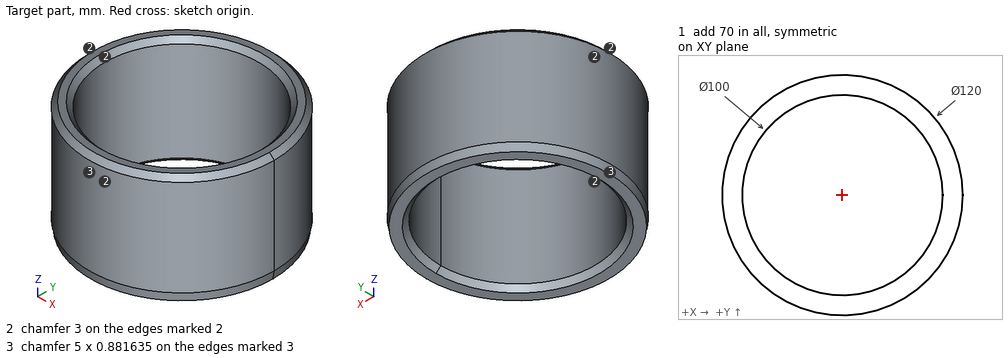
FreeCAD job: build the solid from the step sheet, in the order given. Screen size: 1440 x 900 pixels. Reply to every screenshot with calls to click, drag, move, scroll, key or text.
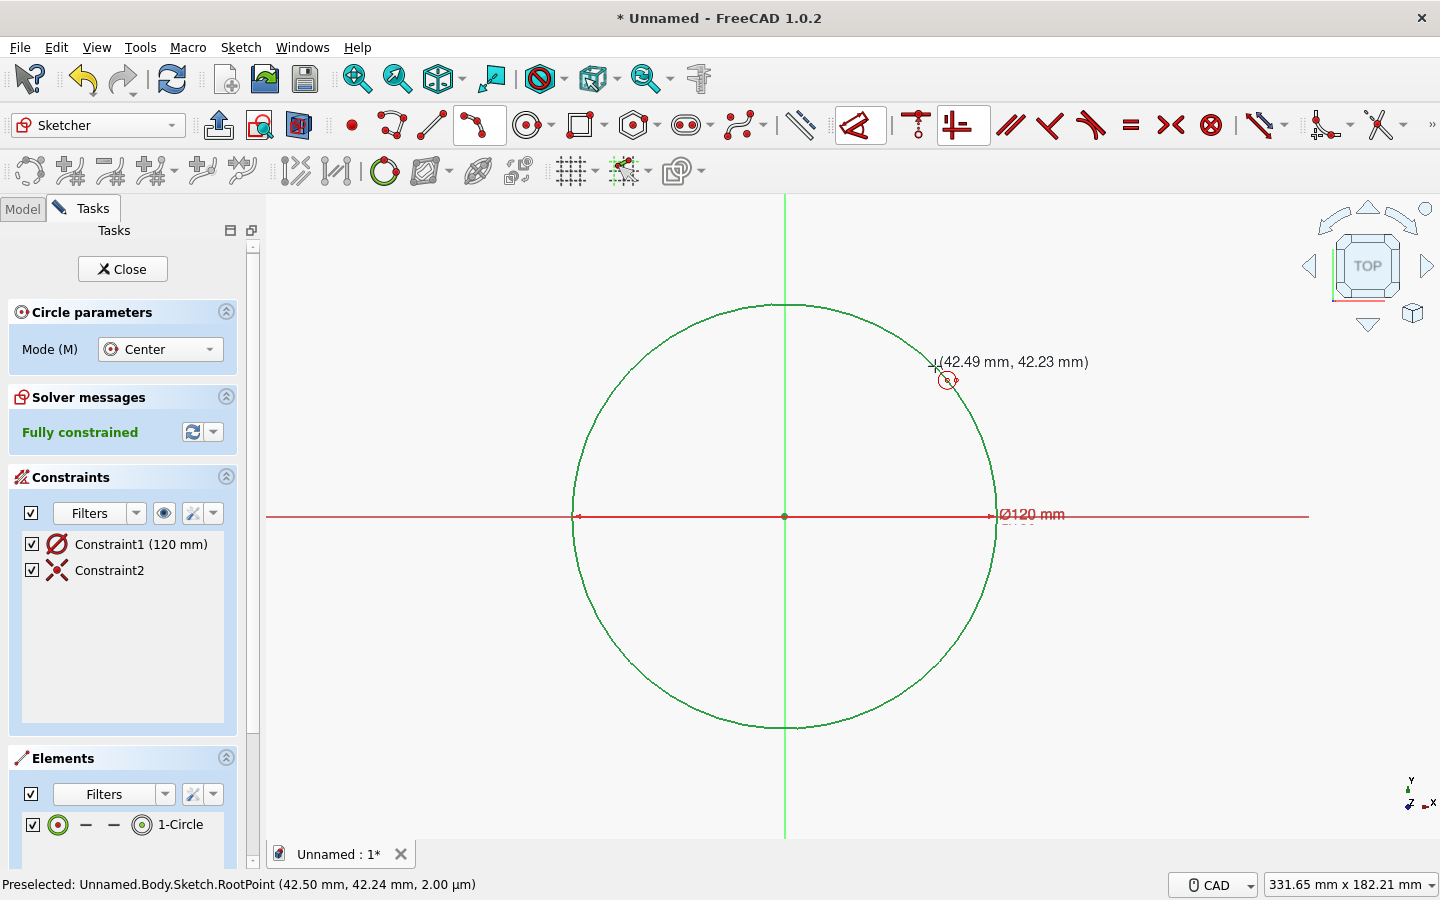
click(785, 516)
move(910, 391)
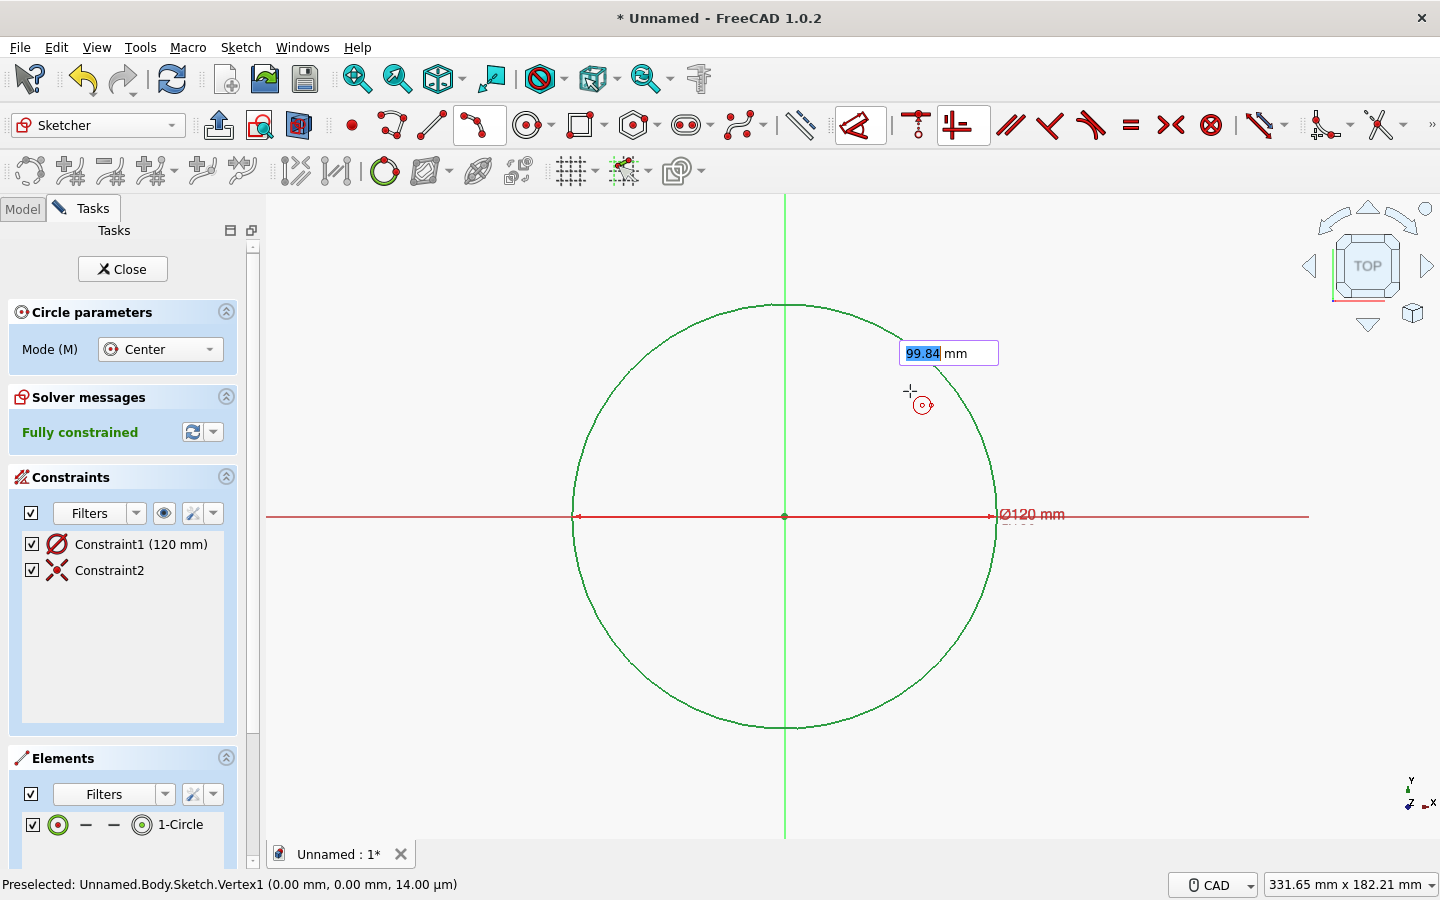
text(100)
key(Return)
key(Escape)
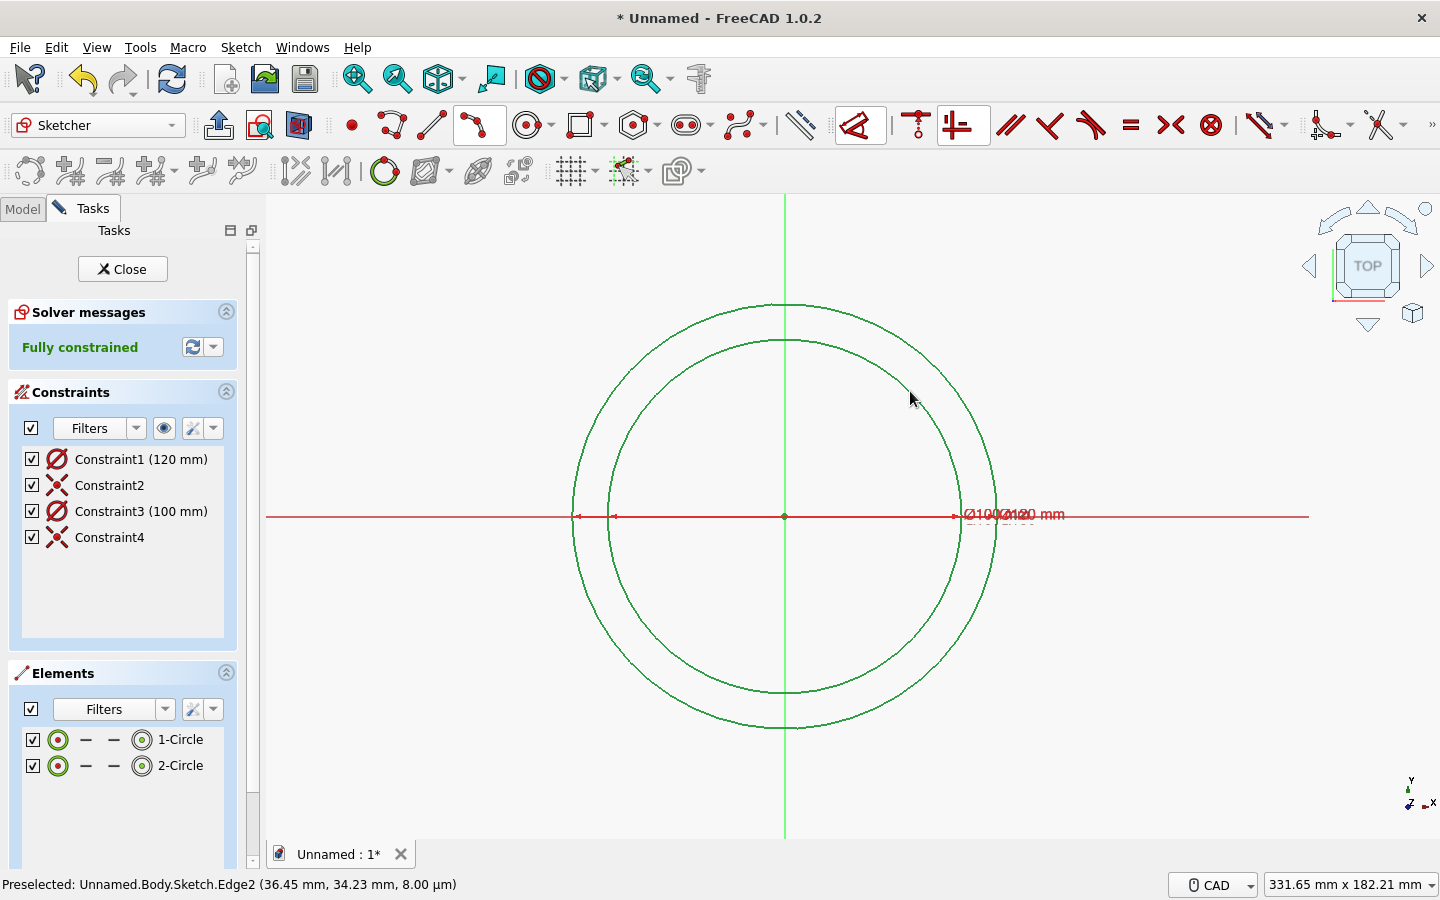
click(123, 269)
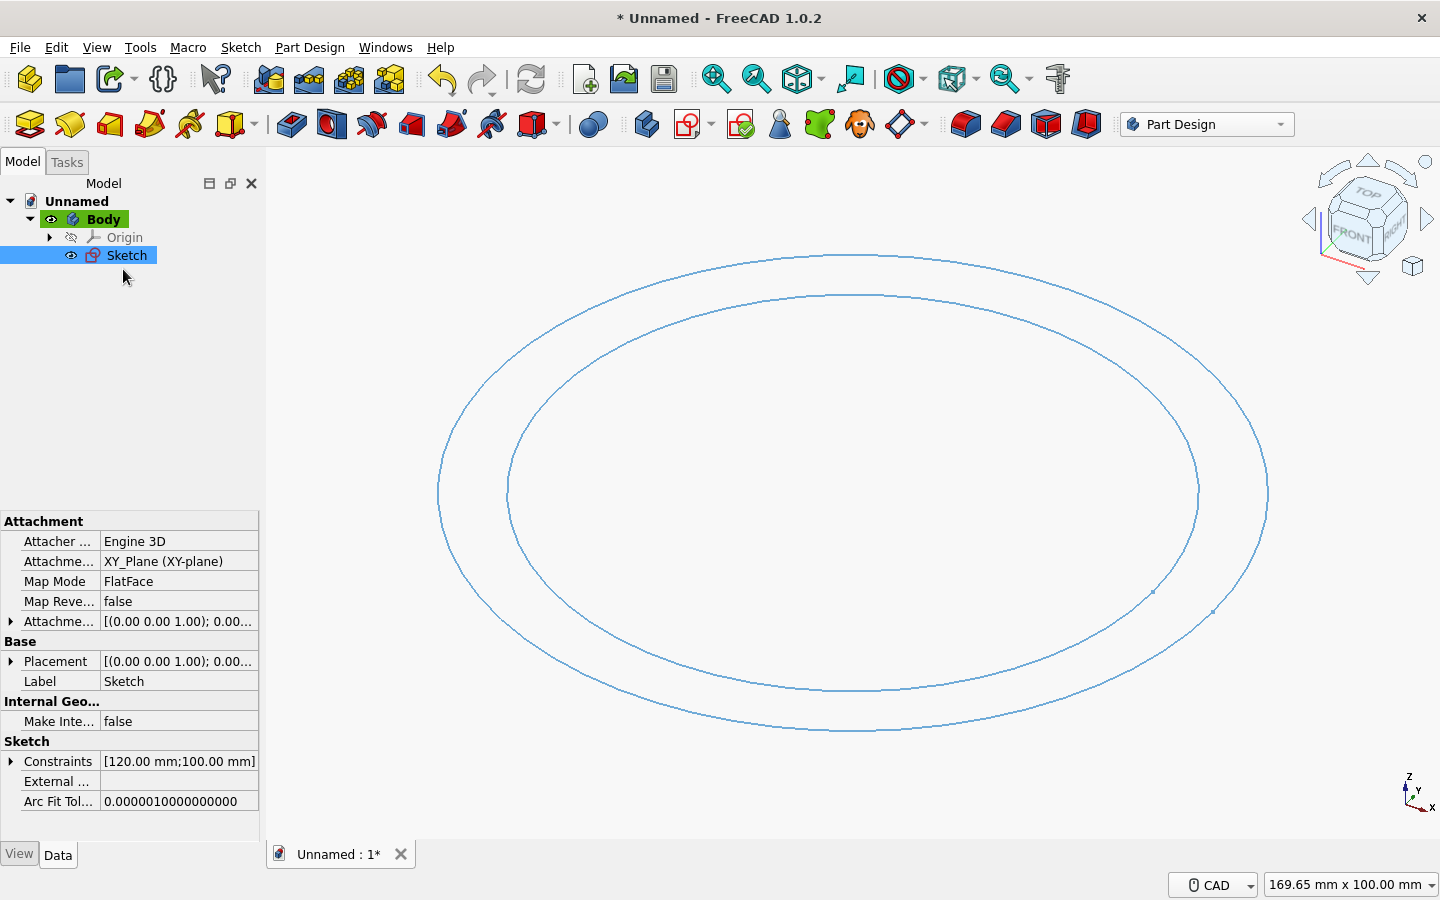
click(30, 124)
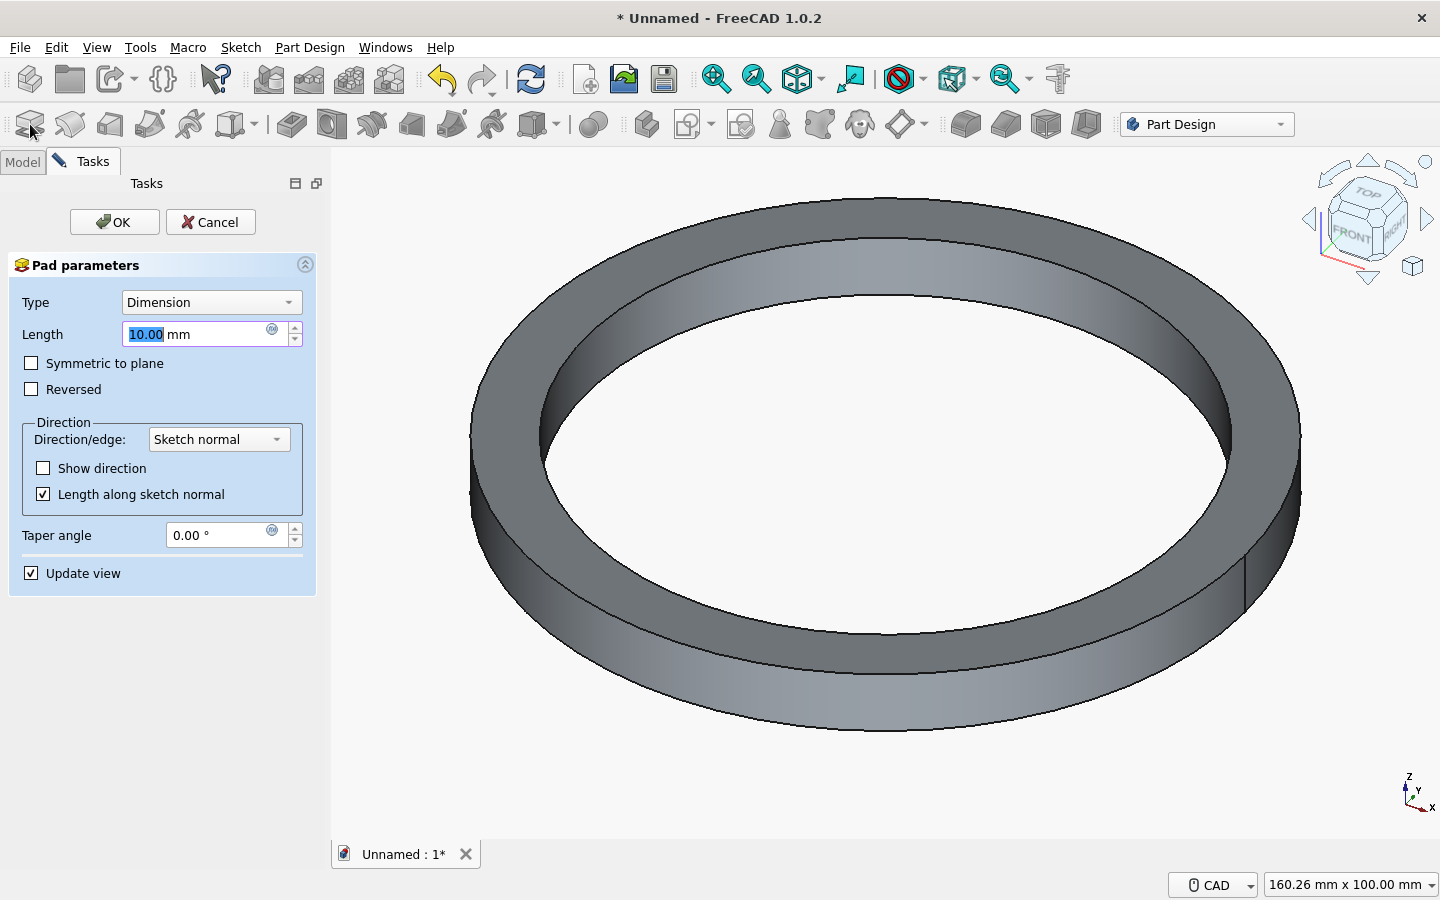
text(70)
key(Tab)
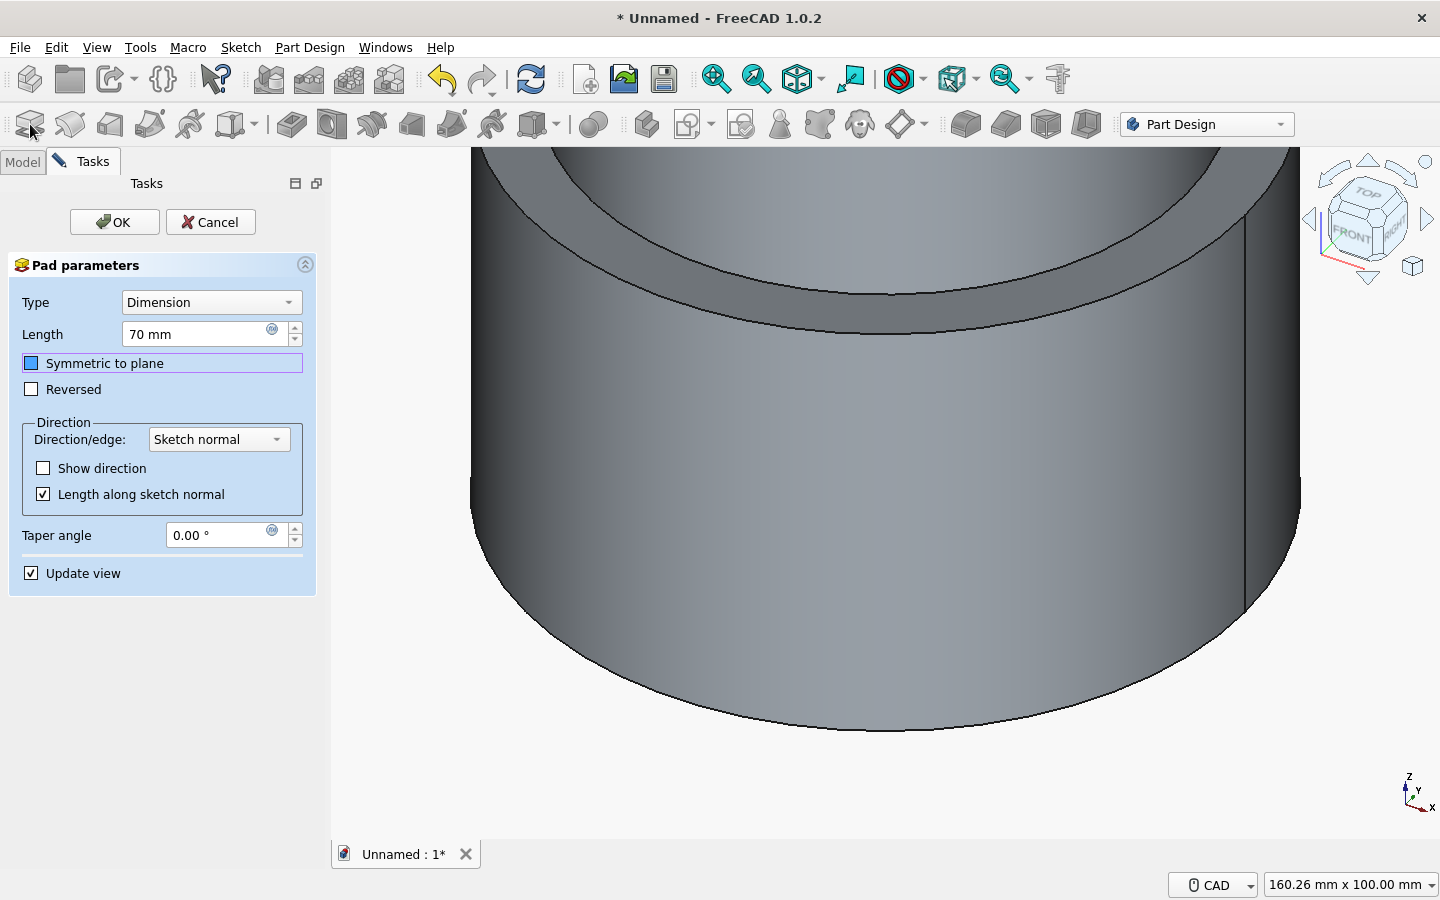
click(30, 363)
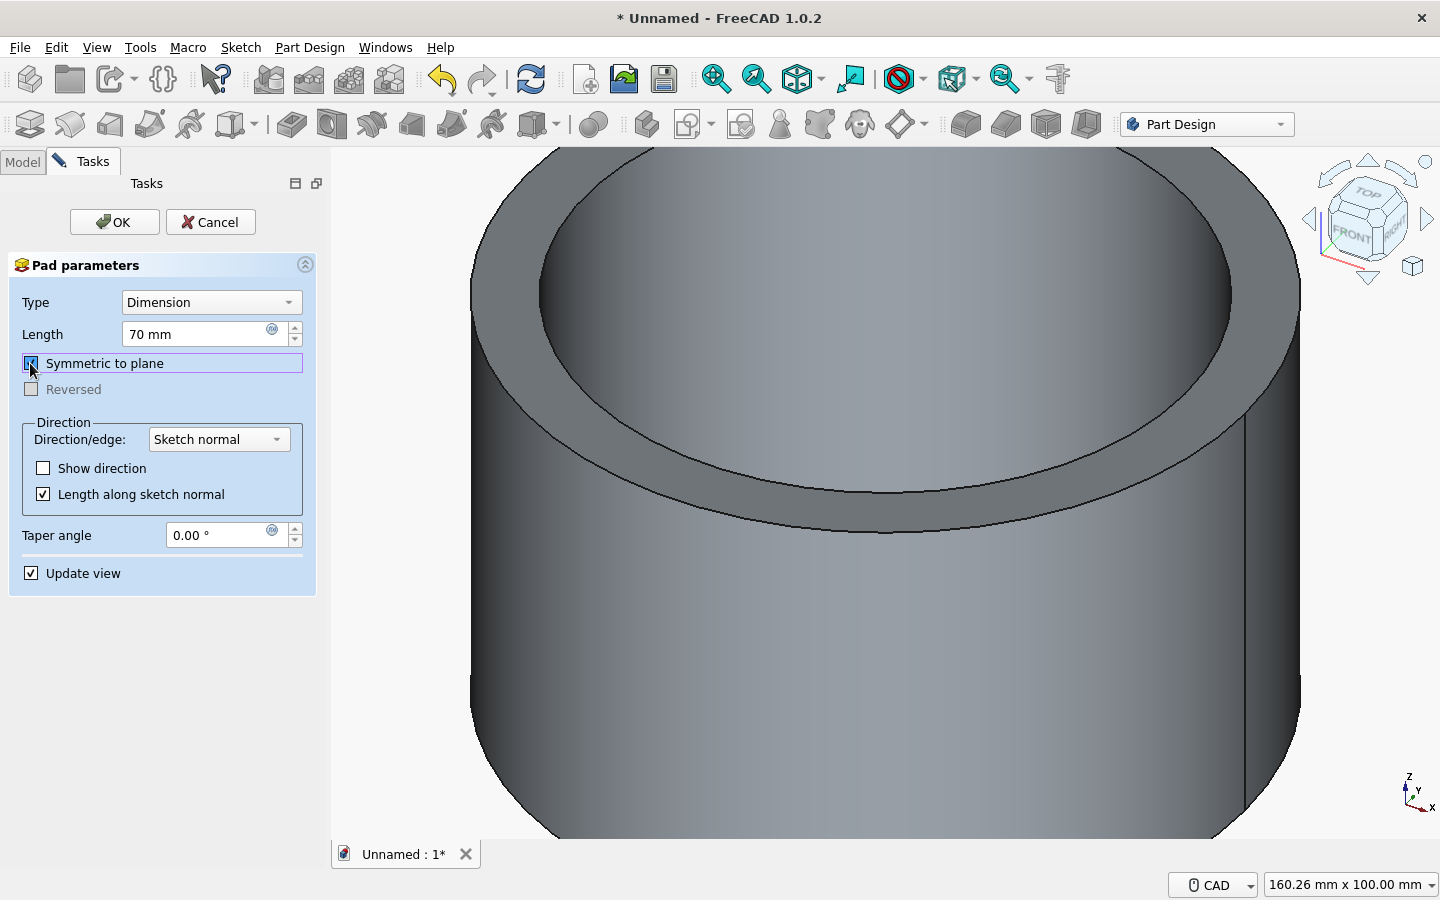
click(115, 222)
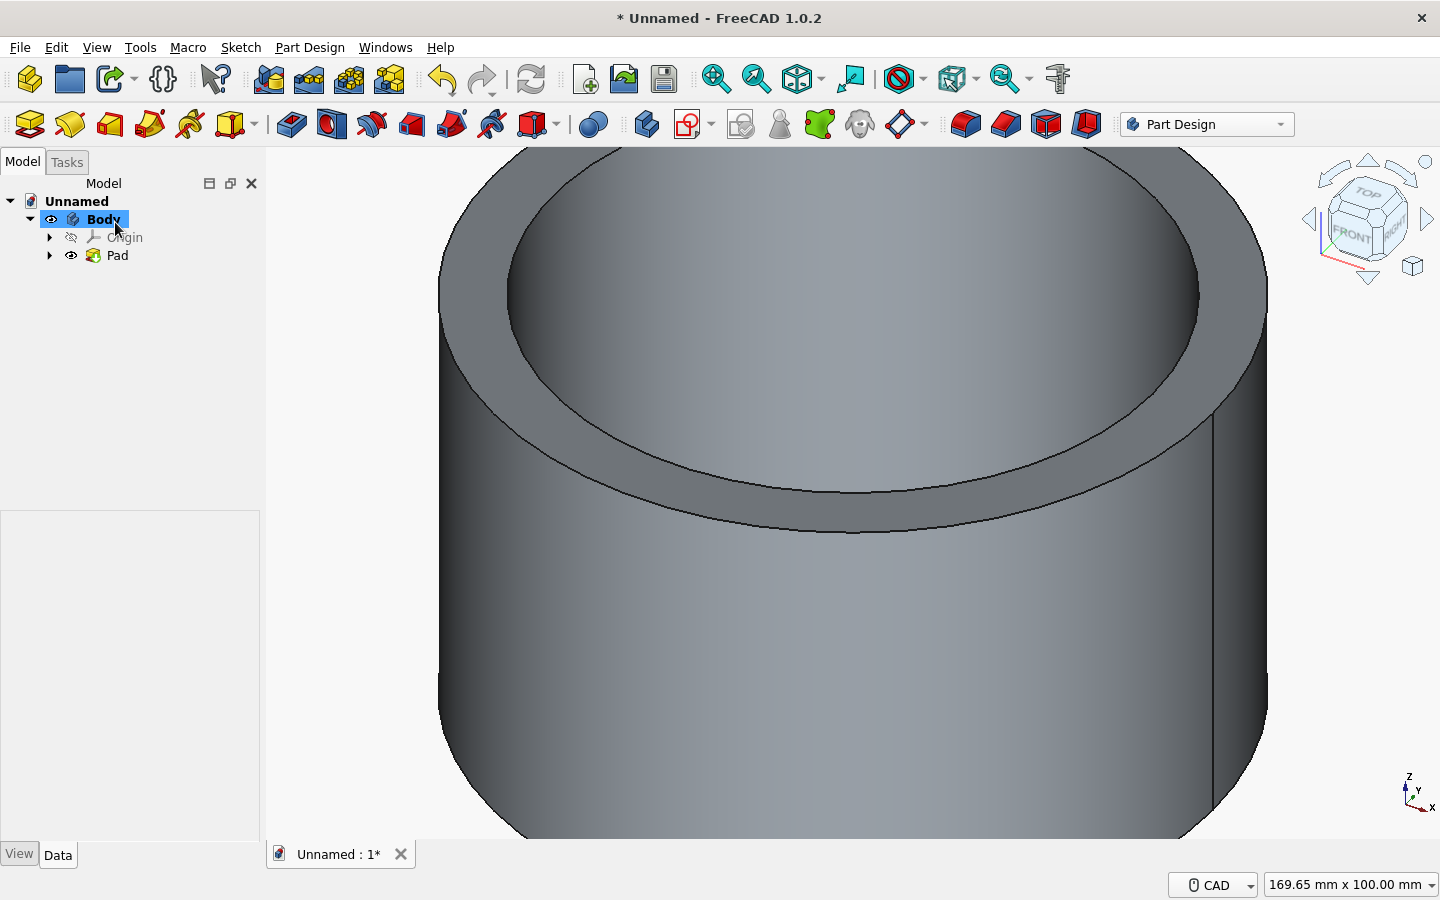
click(718, 80)